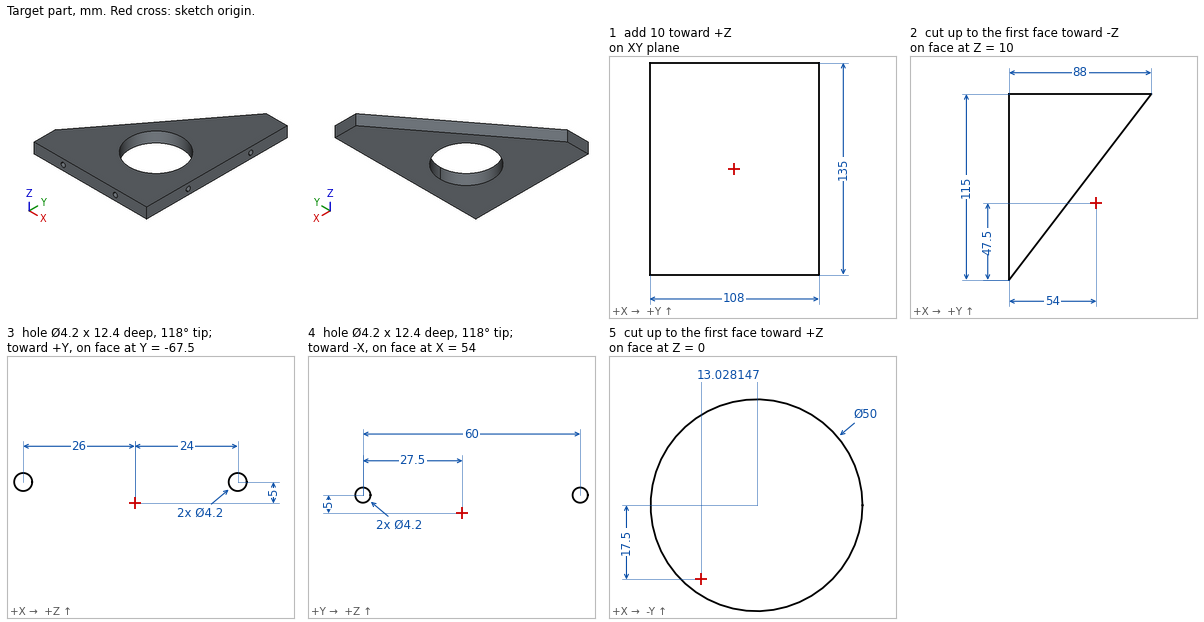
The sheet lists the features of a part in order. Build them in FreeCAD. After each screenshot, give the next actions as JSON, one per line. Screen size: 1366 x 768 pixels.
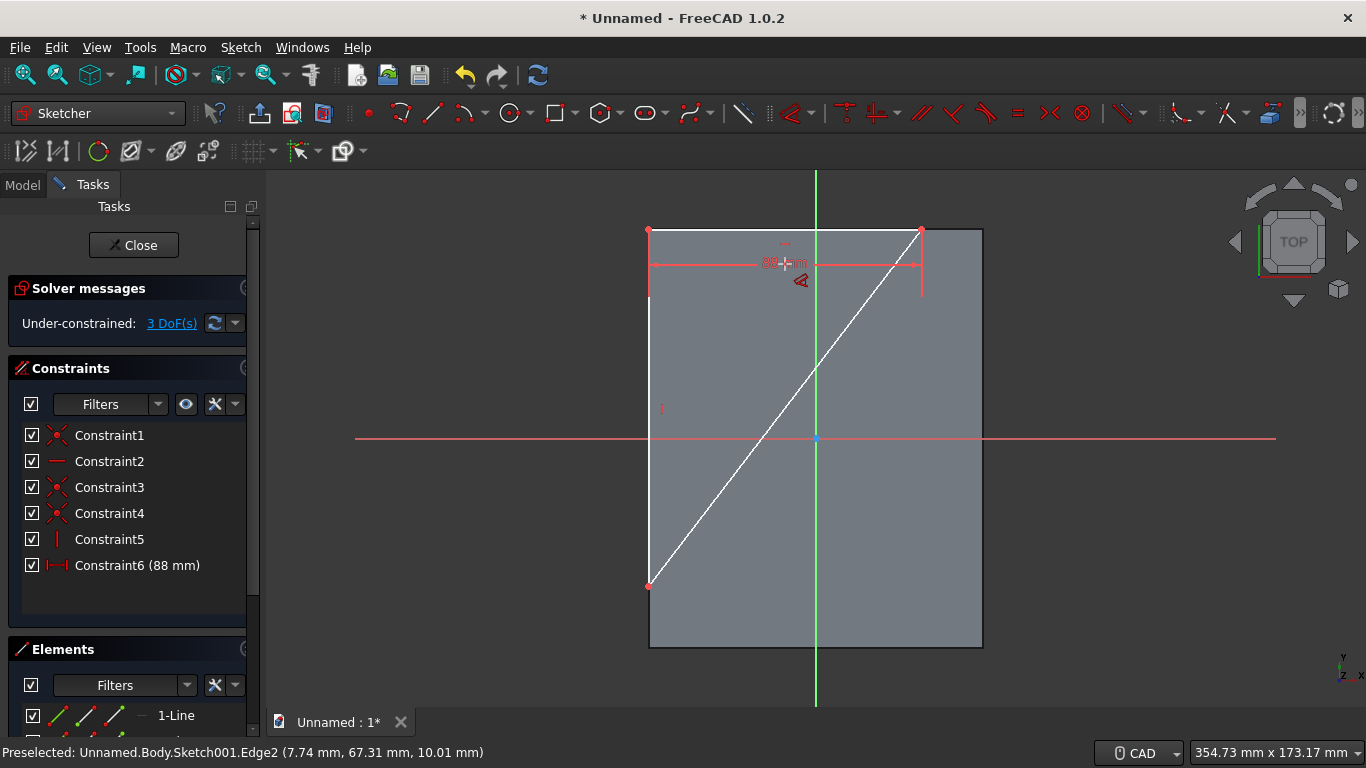
{"action": "left_click", "coordinate": [649, 337]}
{"action": "left_click", "coordinate": [615, 408]}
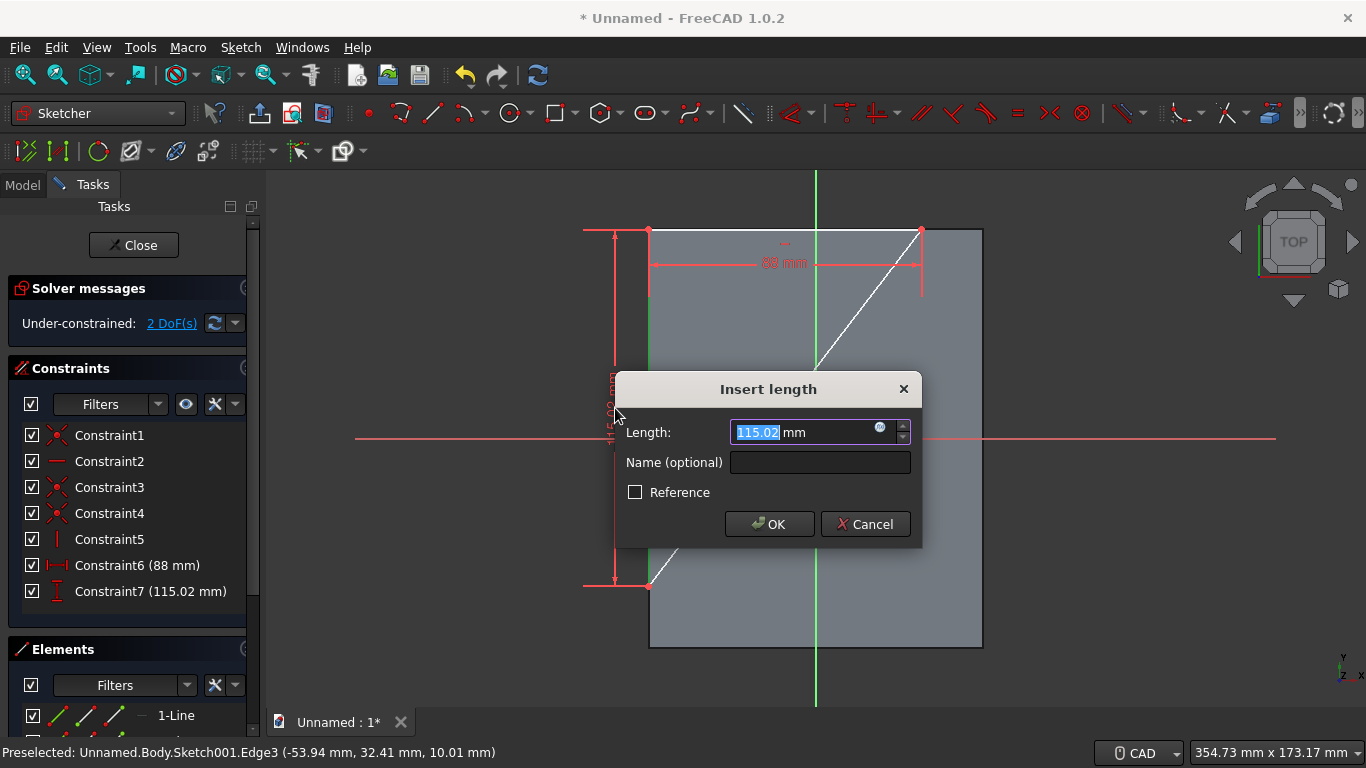
{"action": "type", "text": "115"}
{"action": "key", "text": "Return"}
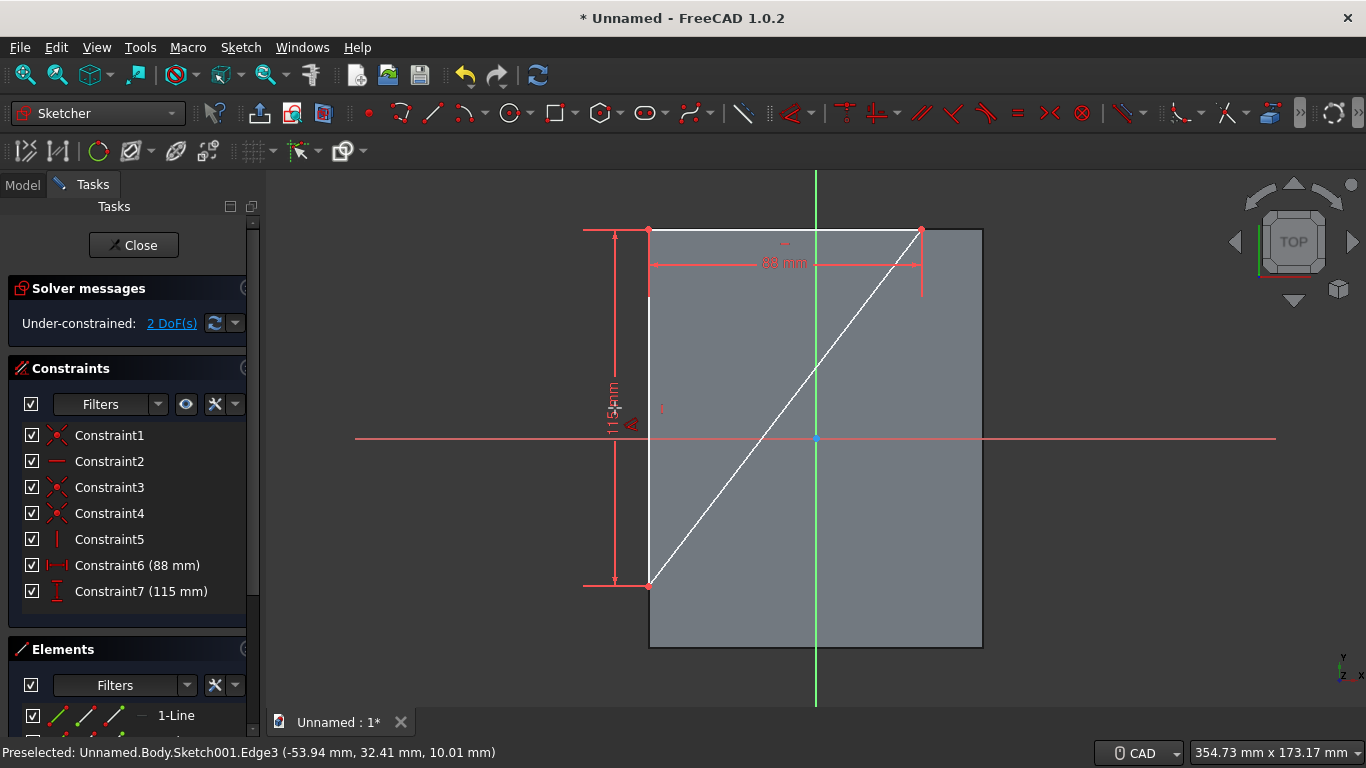
{"action": "left_click", "coordinate": [649, 586]}
{"action": "left_click", "coordinate": [732, 620]}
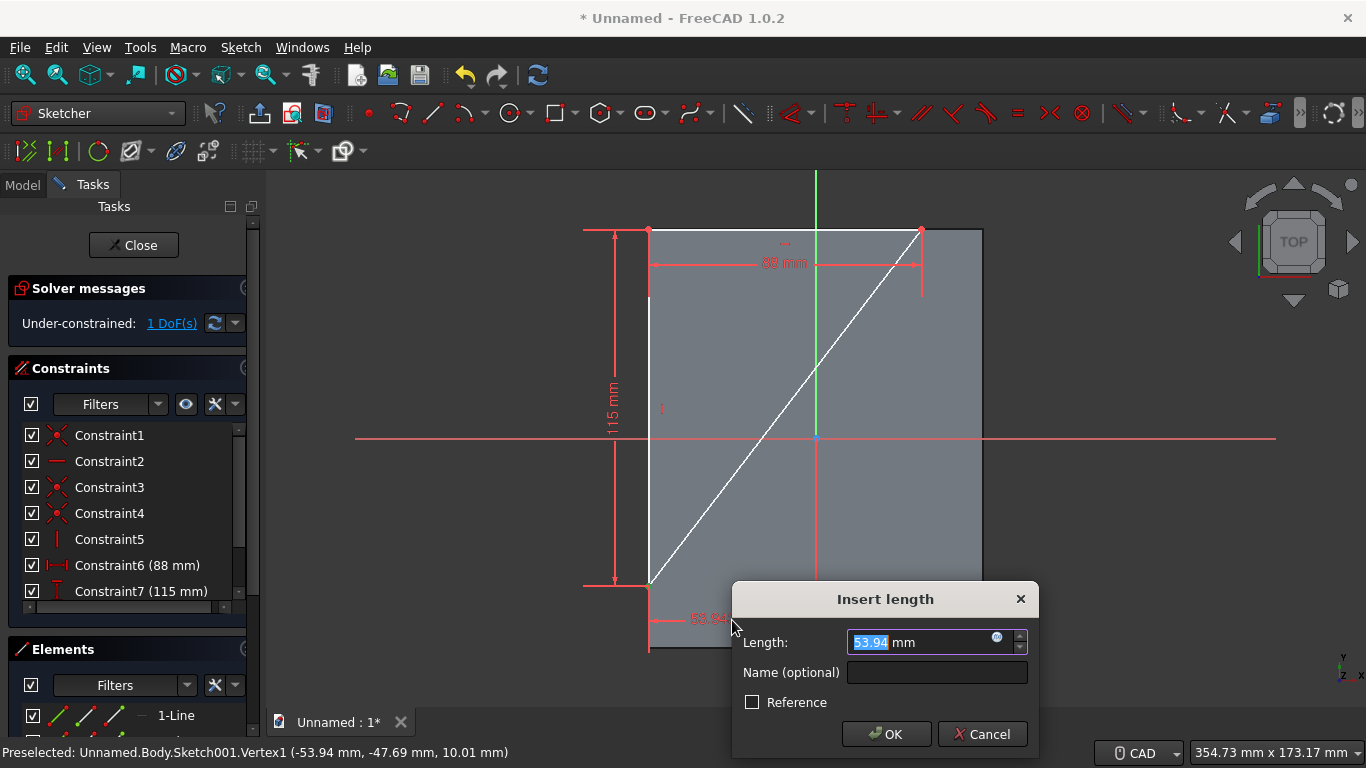
{"action": "type", "text": "54"}
{"action": "key", "text": "Return"}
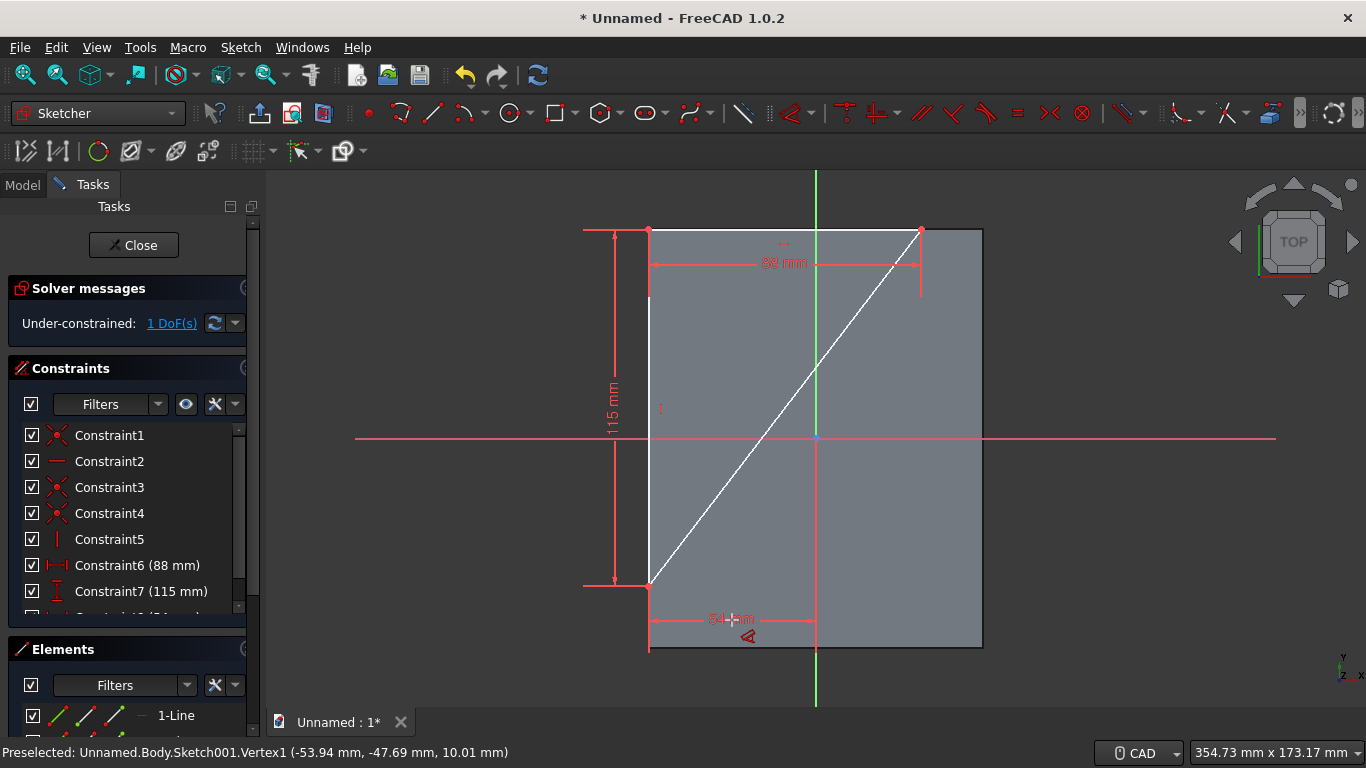
{"action": "left_click", "coordinate": [649, 586]}
{"action": "left_click", "coordinate": [615, 512]}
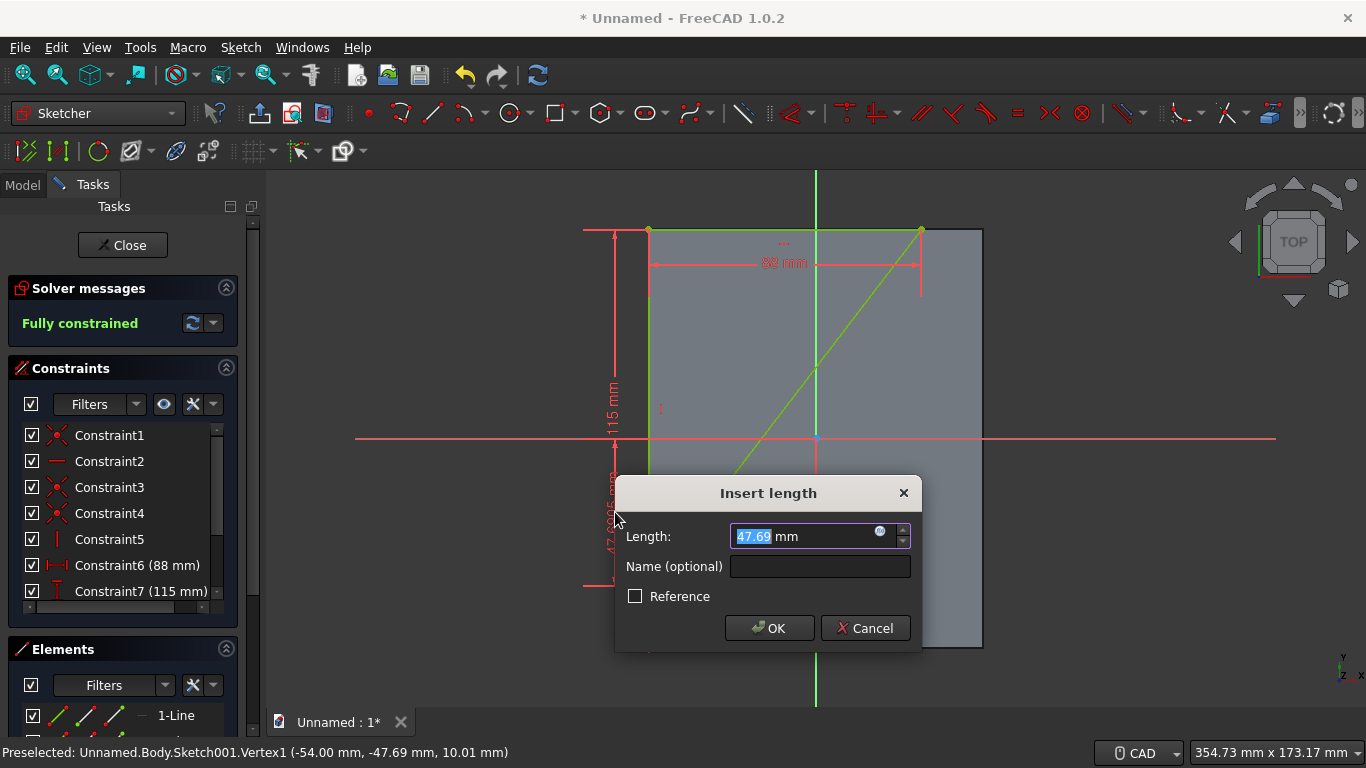
{"action": "type", "text": "47.5"}
{"action": "key", "text": "Return"}
{"action": "key", "text": "Escape"}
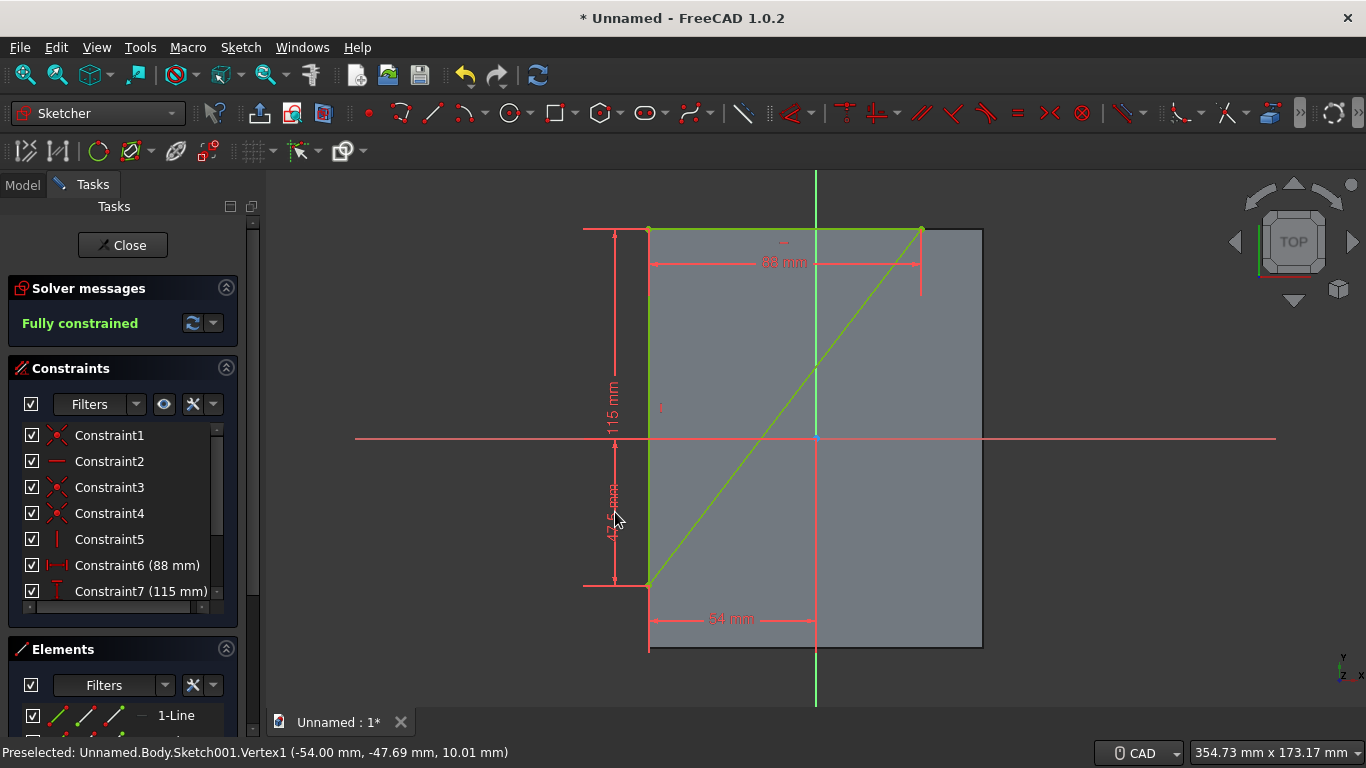
{"action": "left_click", "coordinate": [123, 245]}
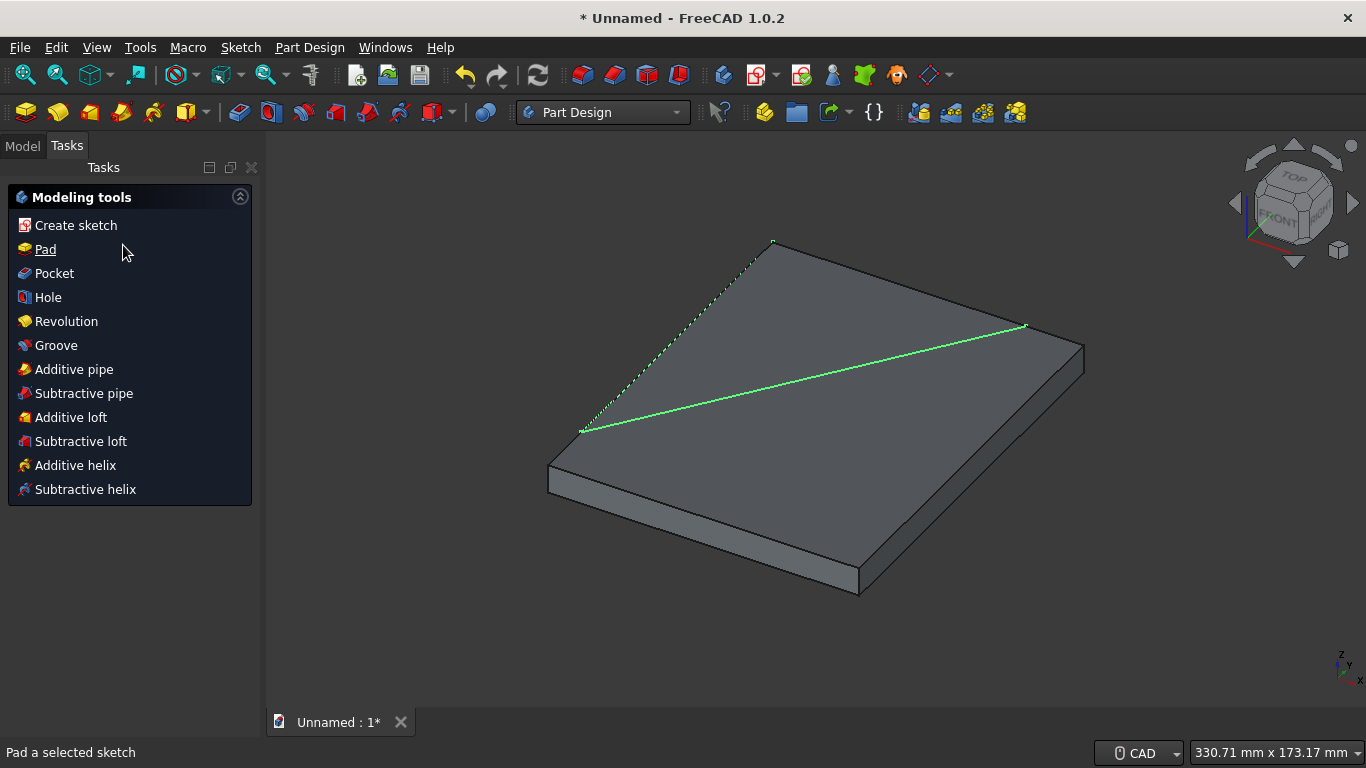
{"action": "left_click", "coordinate": [240, 112]}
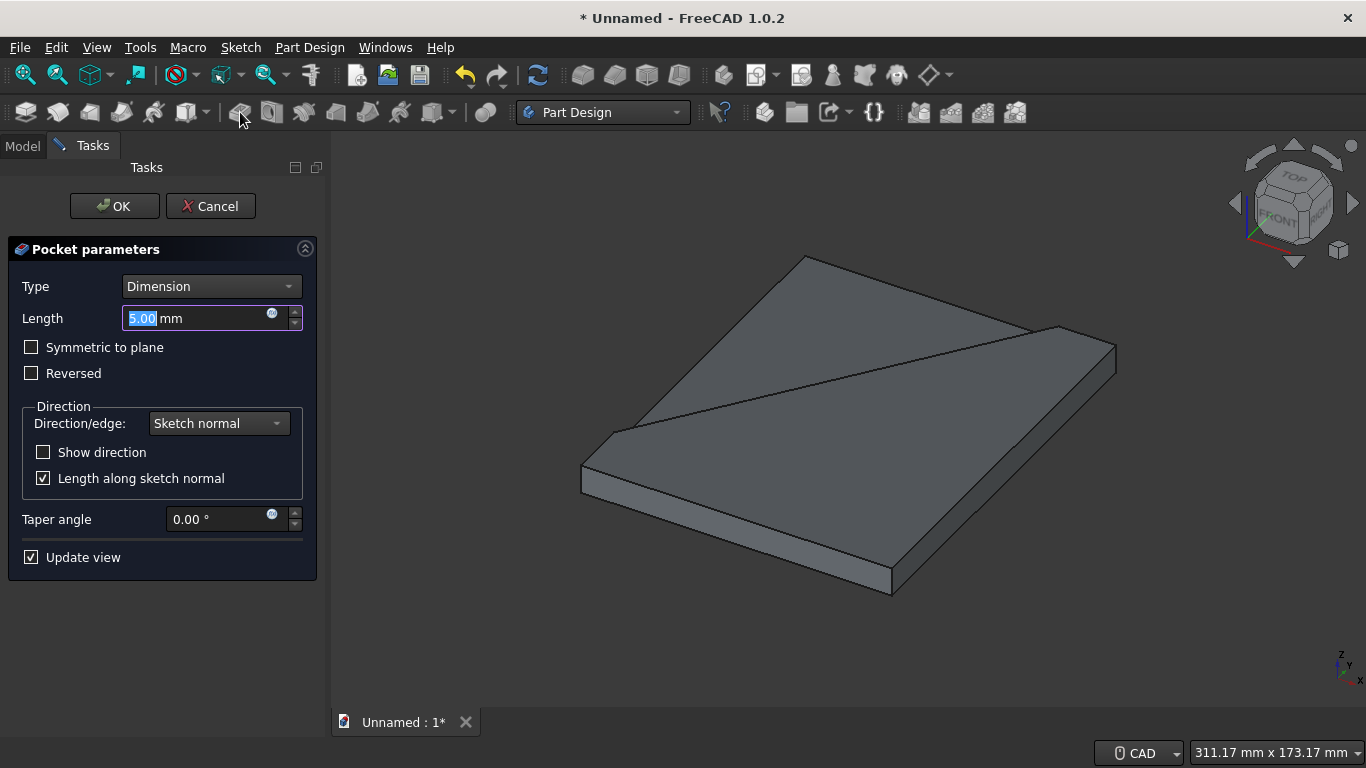
{"action": "left_click", "coordinate": [212, 286]}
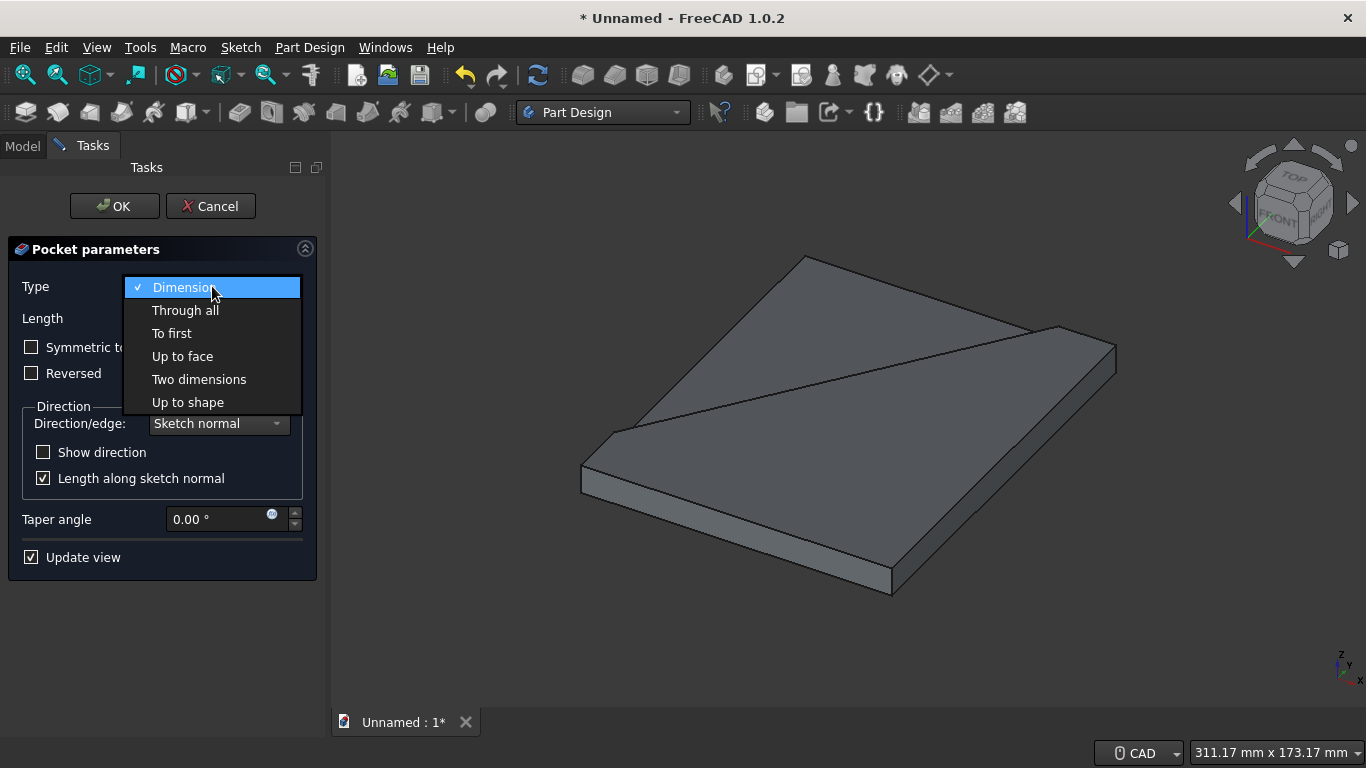
{"action": "left_click", "coordinate": [212, 334]}